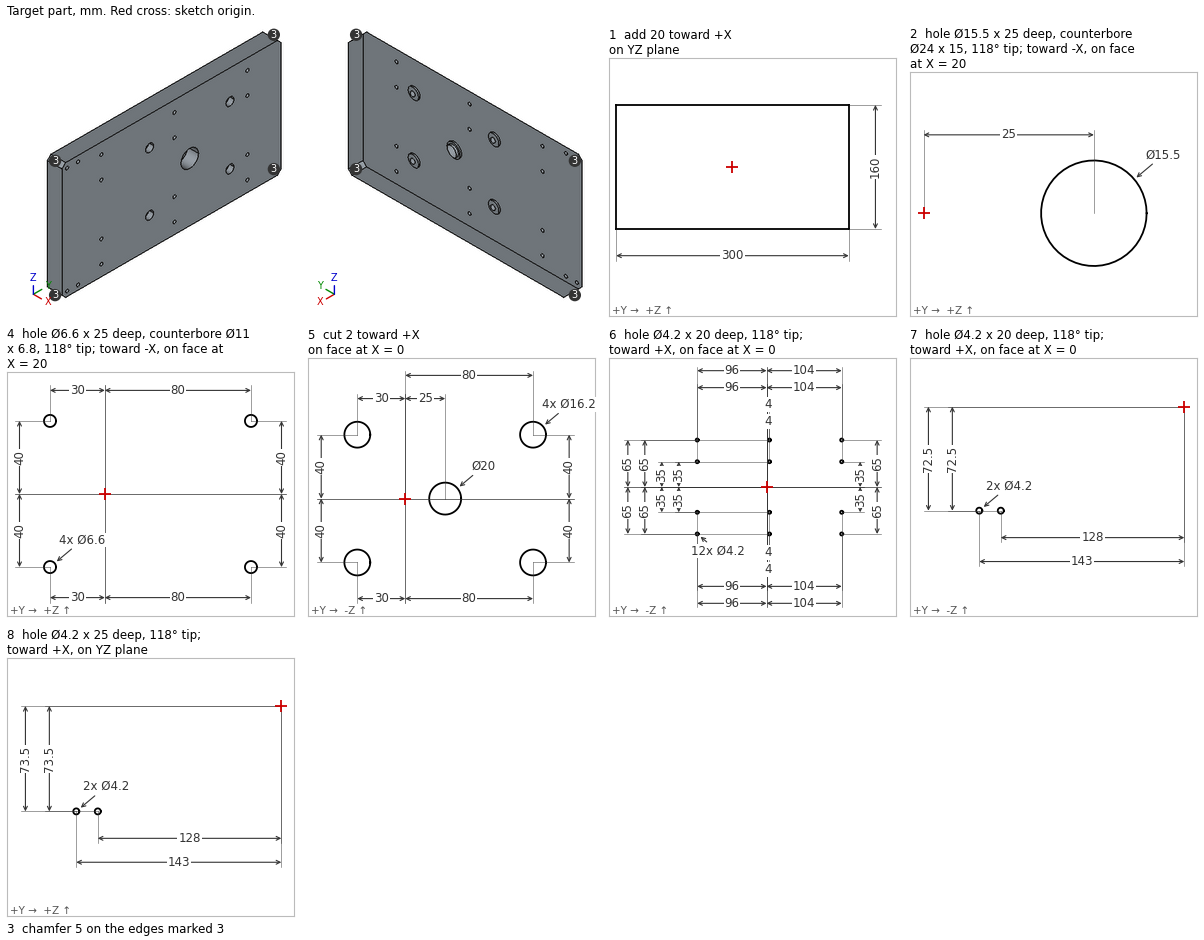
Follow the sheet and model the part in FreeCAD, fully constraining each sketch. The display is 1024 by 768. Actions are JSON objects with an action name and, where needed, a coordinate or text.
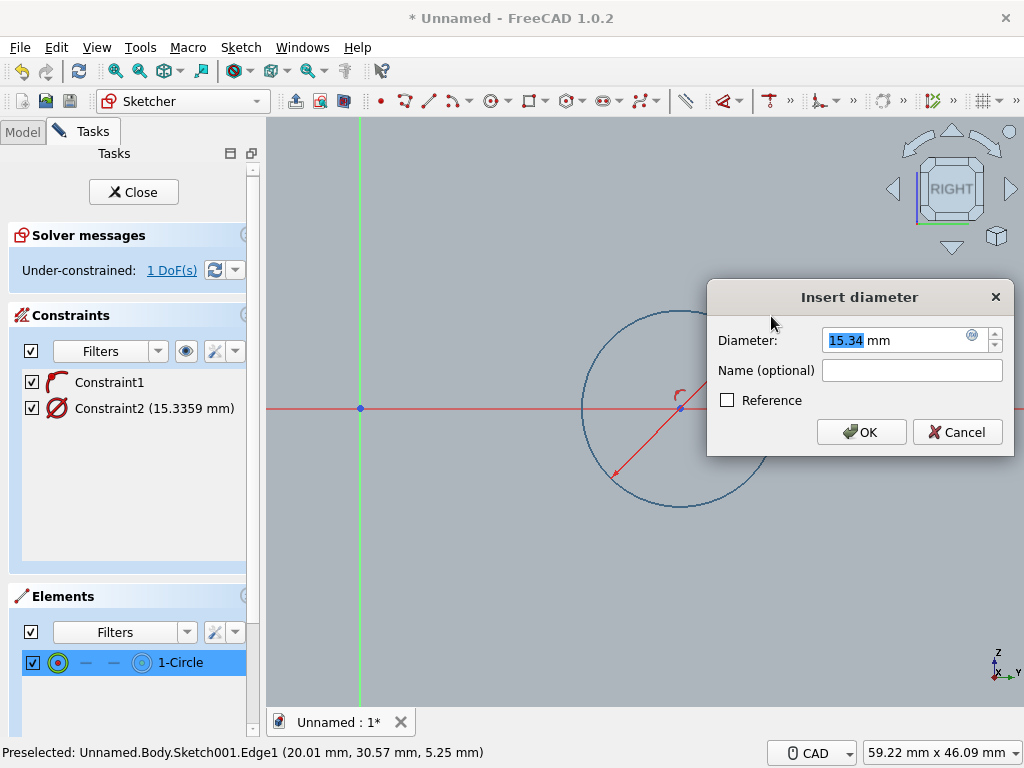
{"action": "type", "text": "15.5"}
{"action": "key", "text": "Return"}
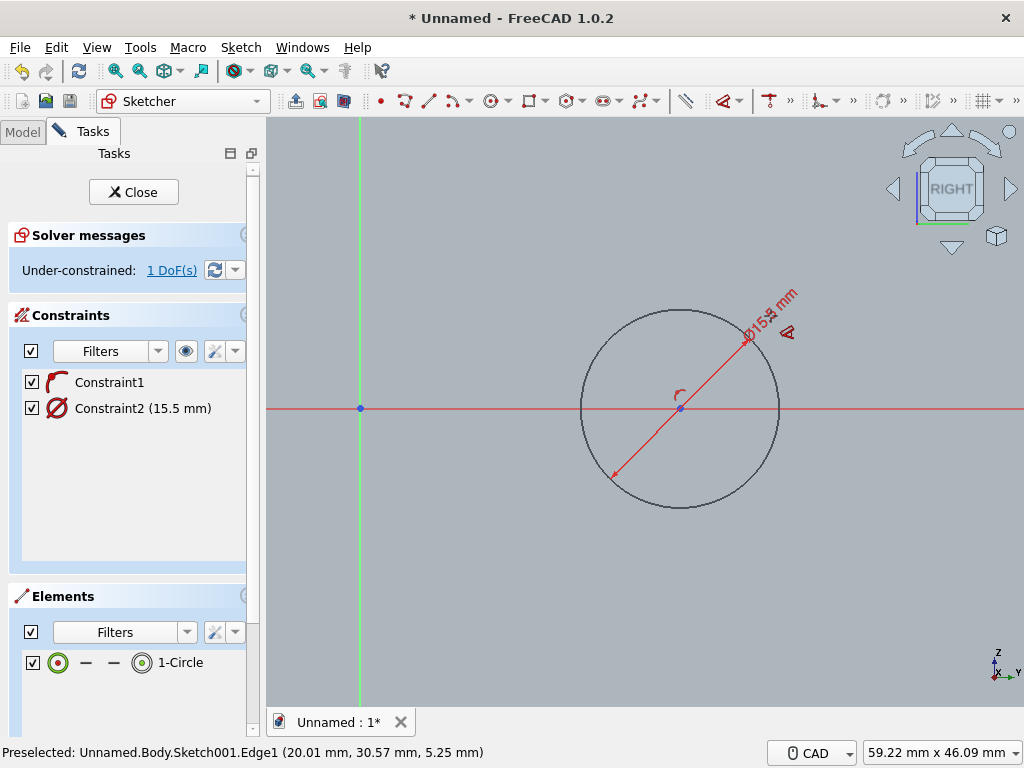
{"action": "left_click", "coordinate": [680, 409]}
{"action": "left_click", "coordinate": [520, 443]}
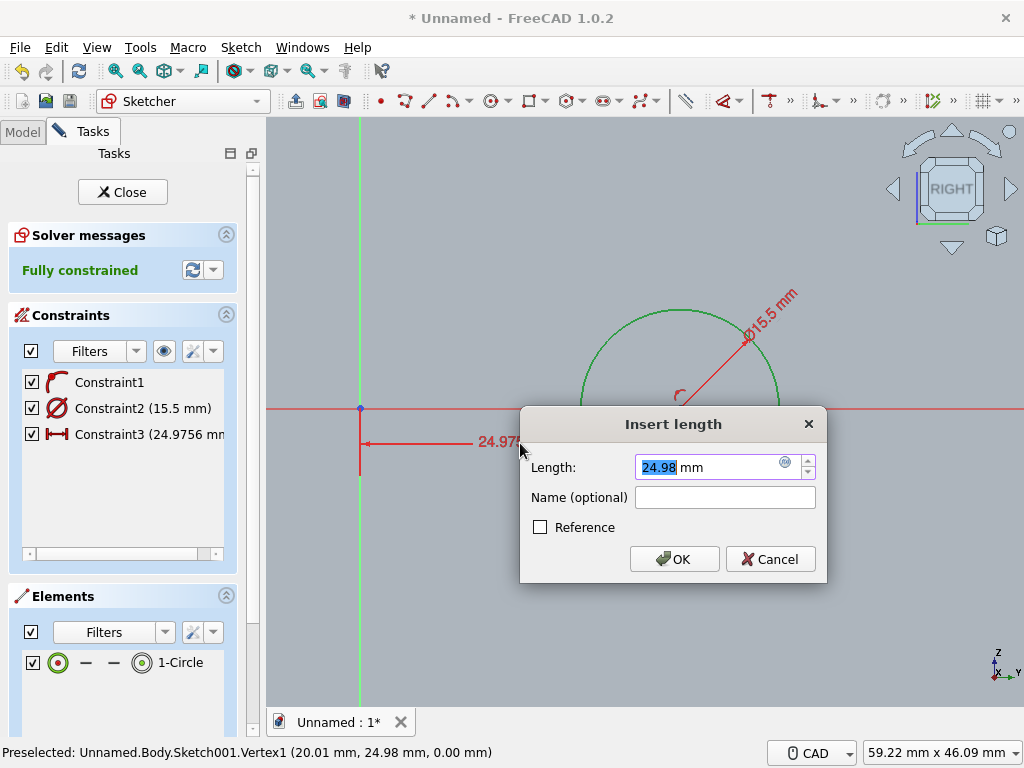
{"action": "type", "text": "25"}
{"action": "key", "text": "Return"}
{"action": "key", "text": "Escape"}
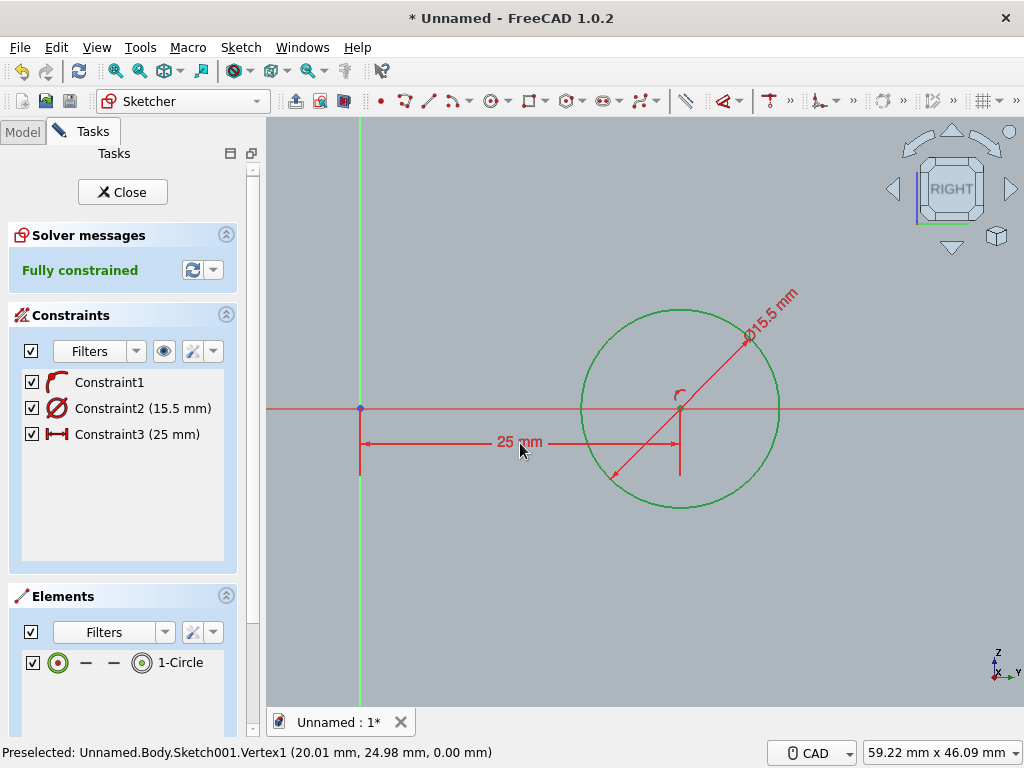
{"action": "left_click", "coordinate": [123, 192]}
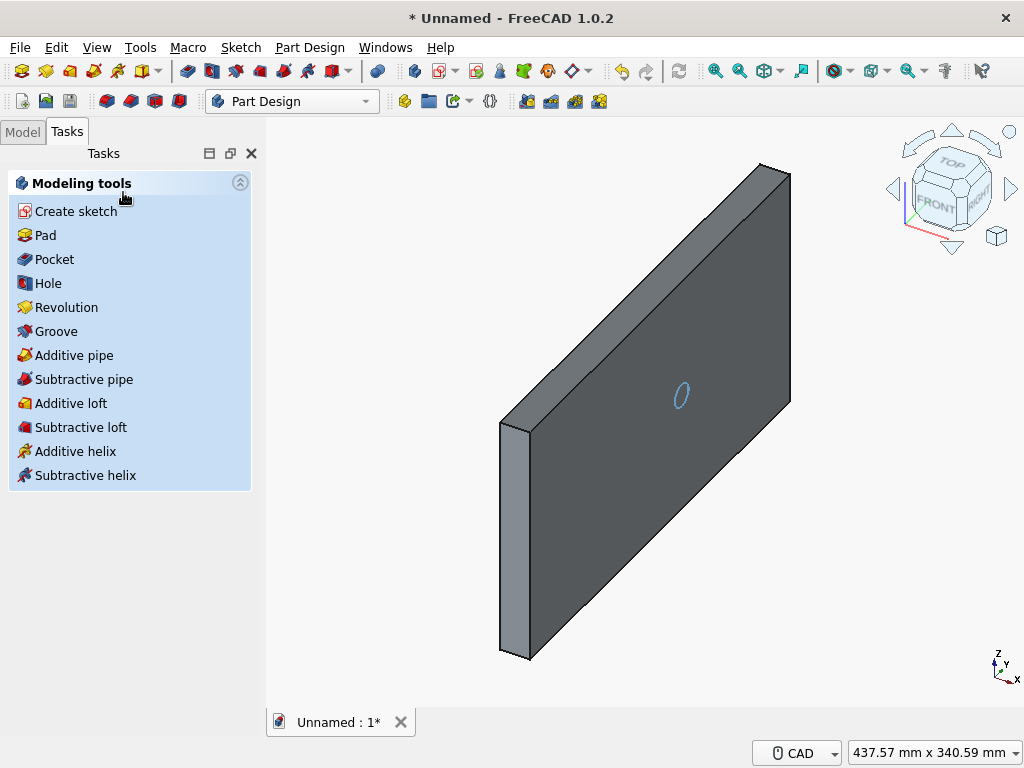
{"action": "left_click", "coordinate": [212, 72]}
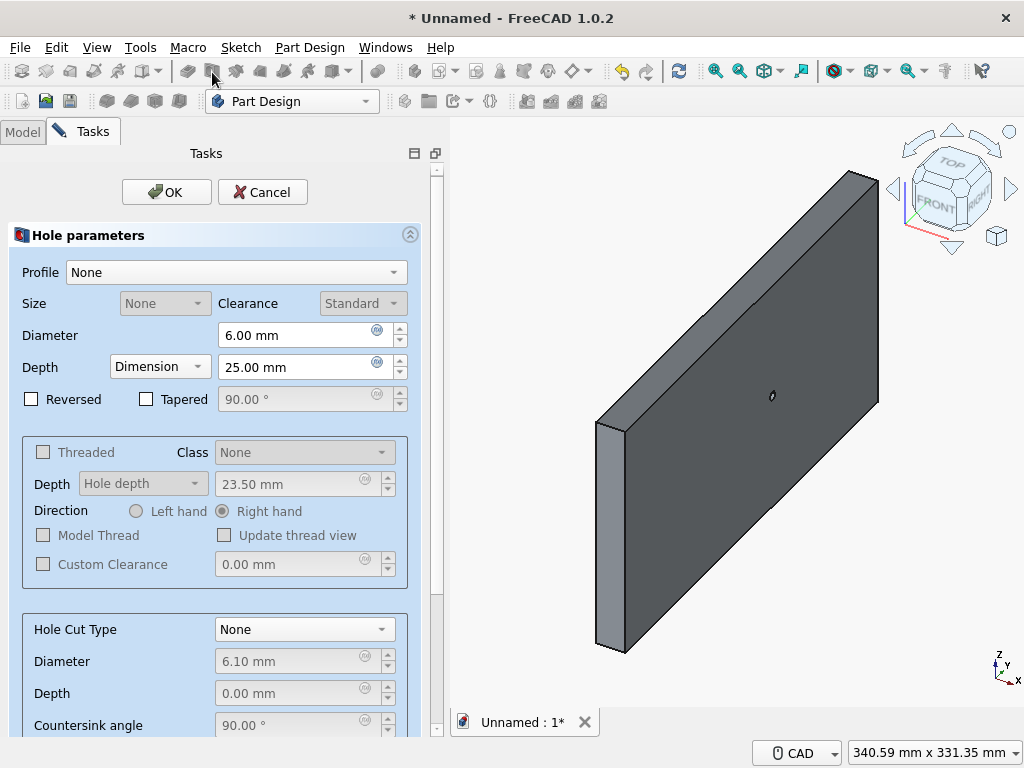
{"action": "triple_click", "coordinate": [305, 335]}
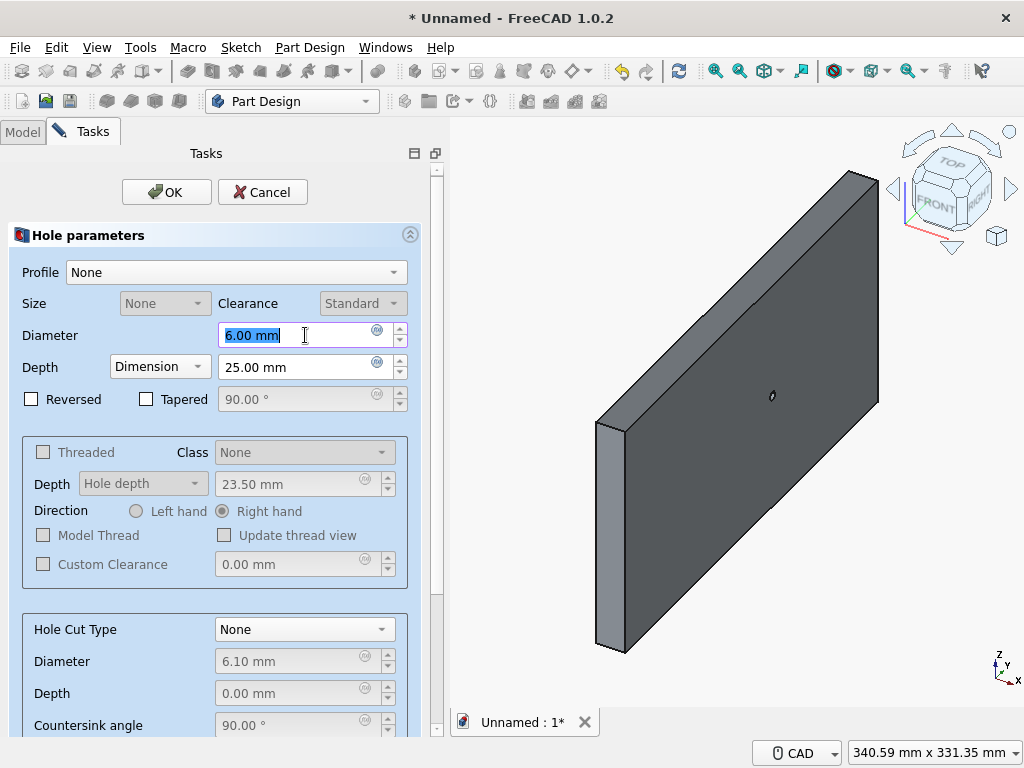
{"action": "type", "text": "15.5"}
{"action": "key", "text": "Tab"}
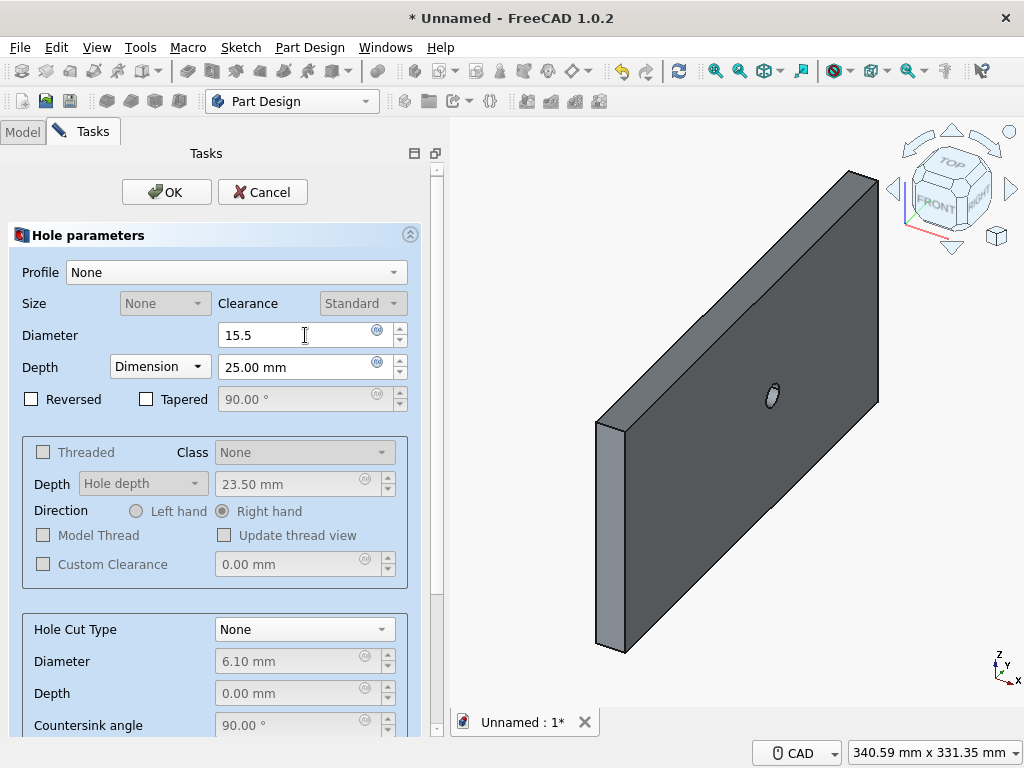
{"action": "triple_click", "coordinate": [305, 367]}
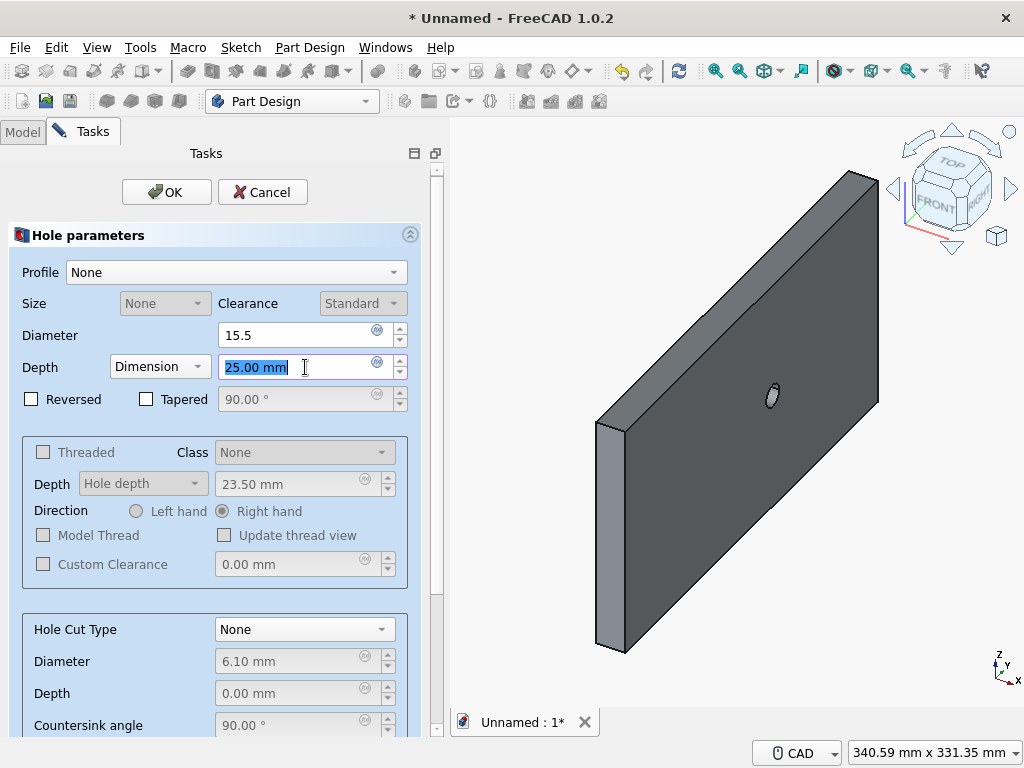
{"action": "type", "text": "25"}
{"action": "key", "text": "Tab"}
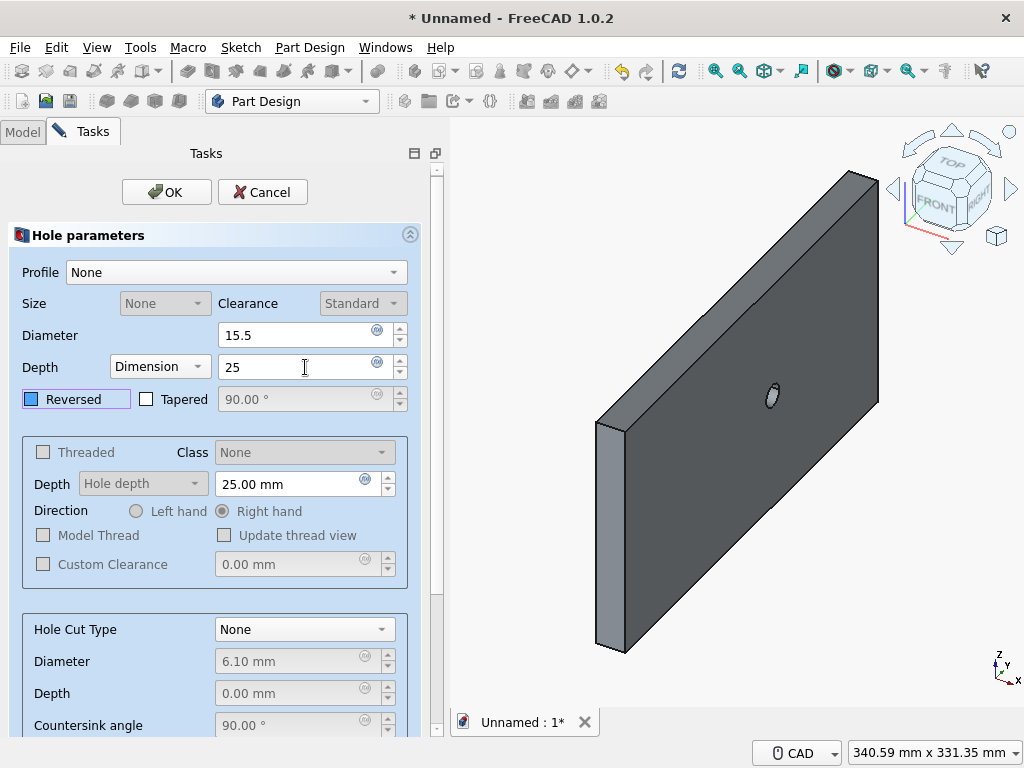
{"action": "left_click", "coordinate": [306, 630]}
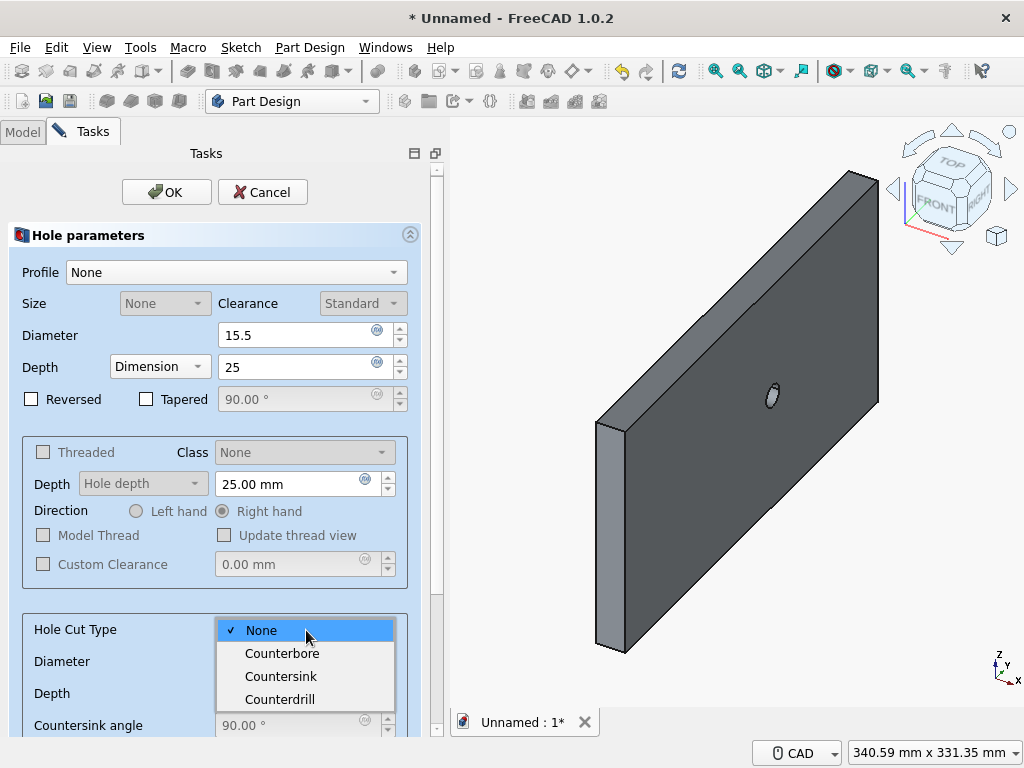
{"action": "left_click", "coordinate": [304, 654]}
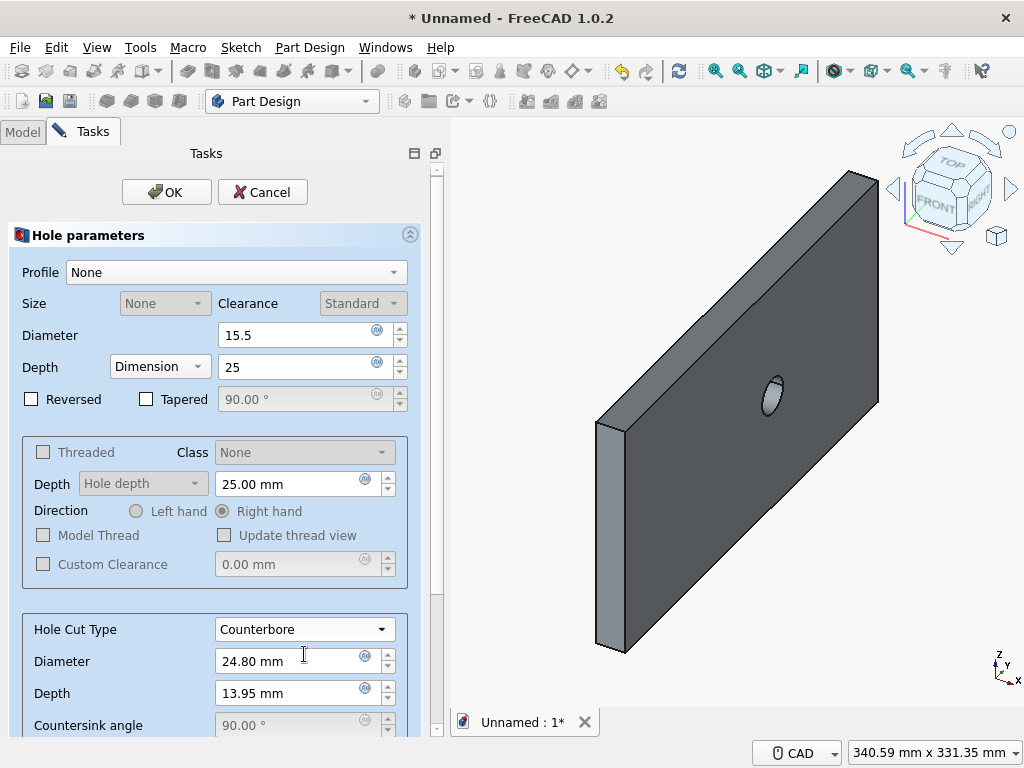
{"action": "triple_click", "coordinate": [298, 661]}